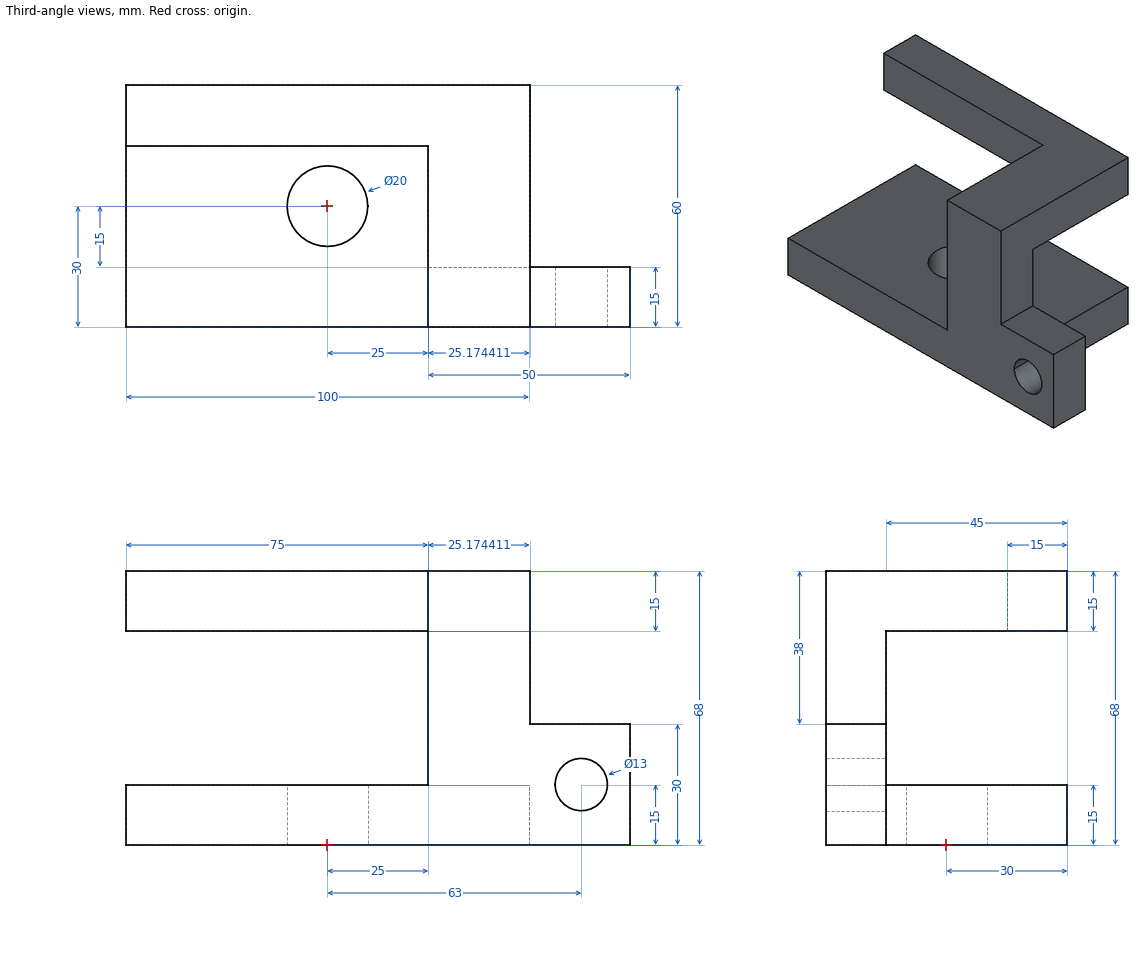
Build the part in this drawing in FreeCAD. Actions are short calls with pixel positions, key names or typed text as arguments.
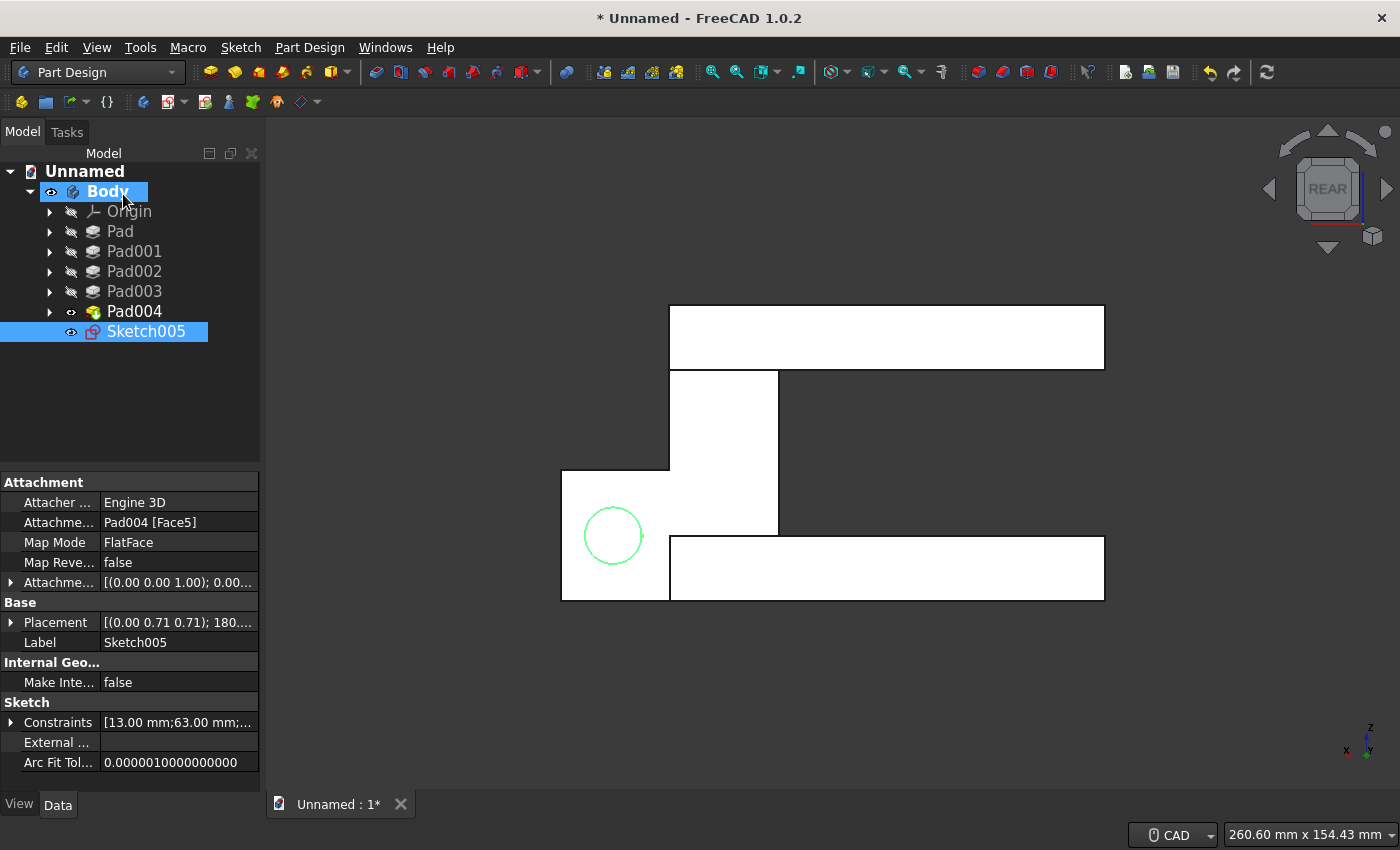
click(378, 72)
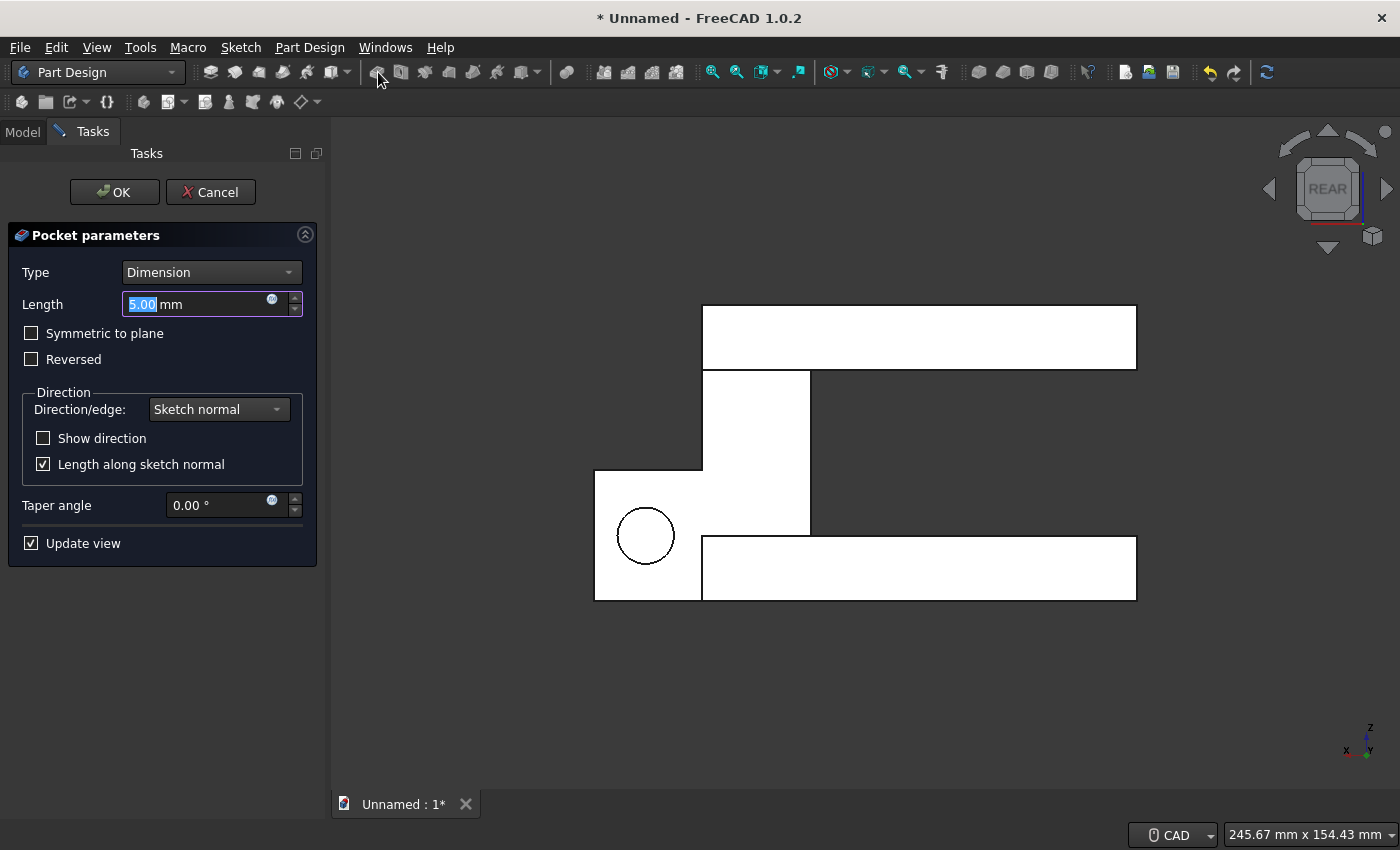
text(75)
key(Tab)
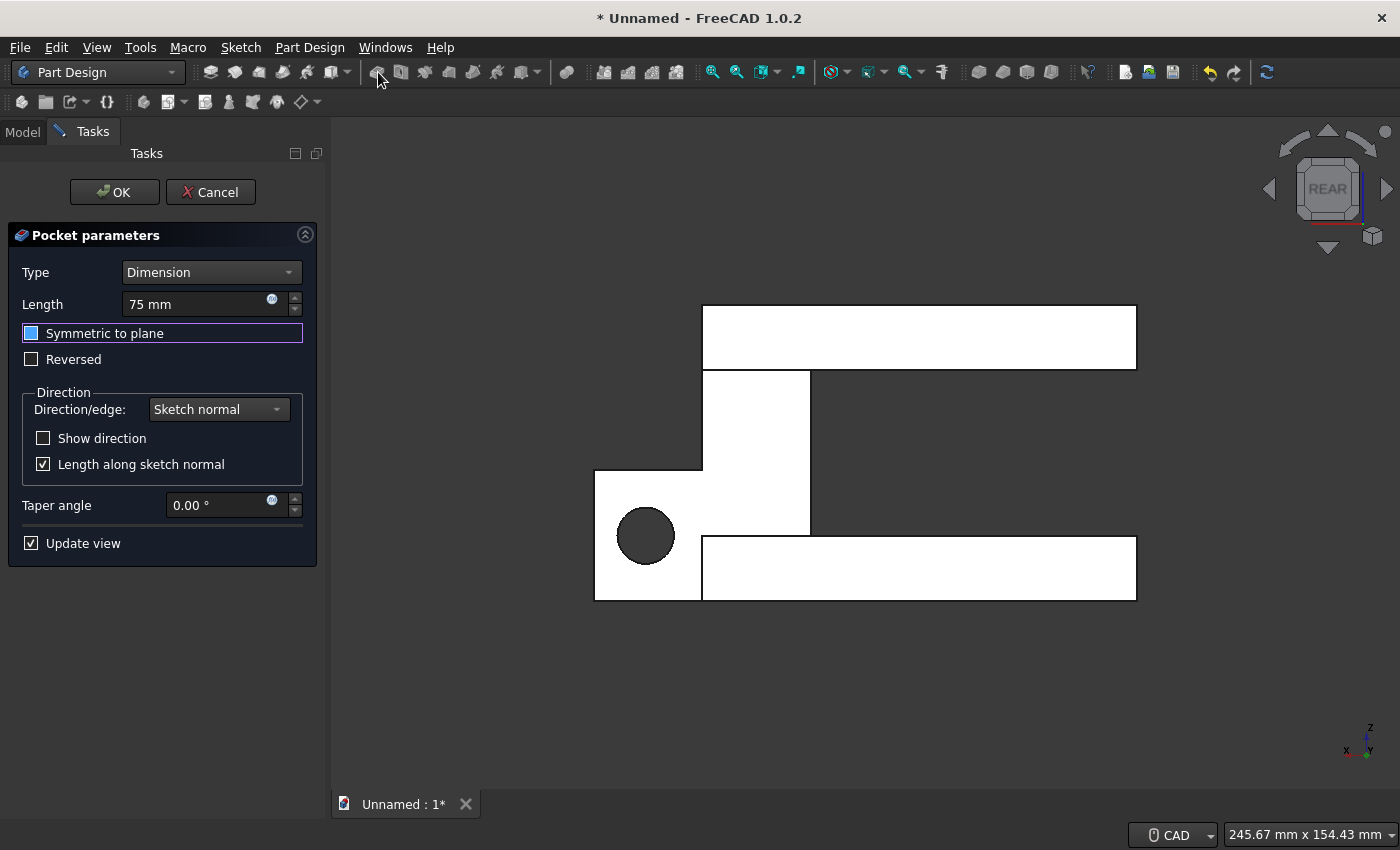
click(115, 192)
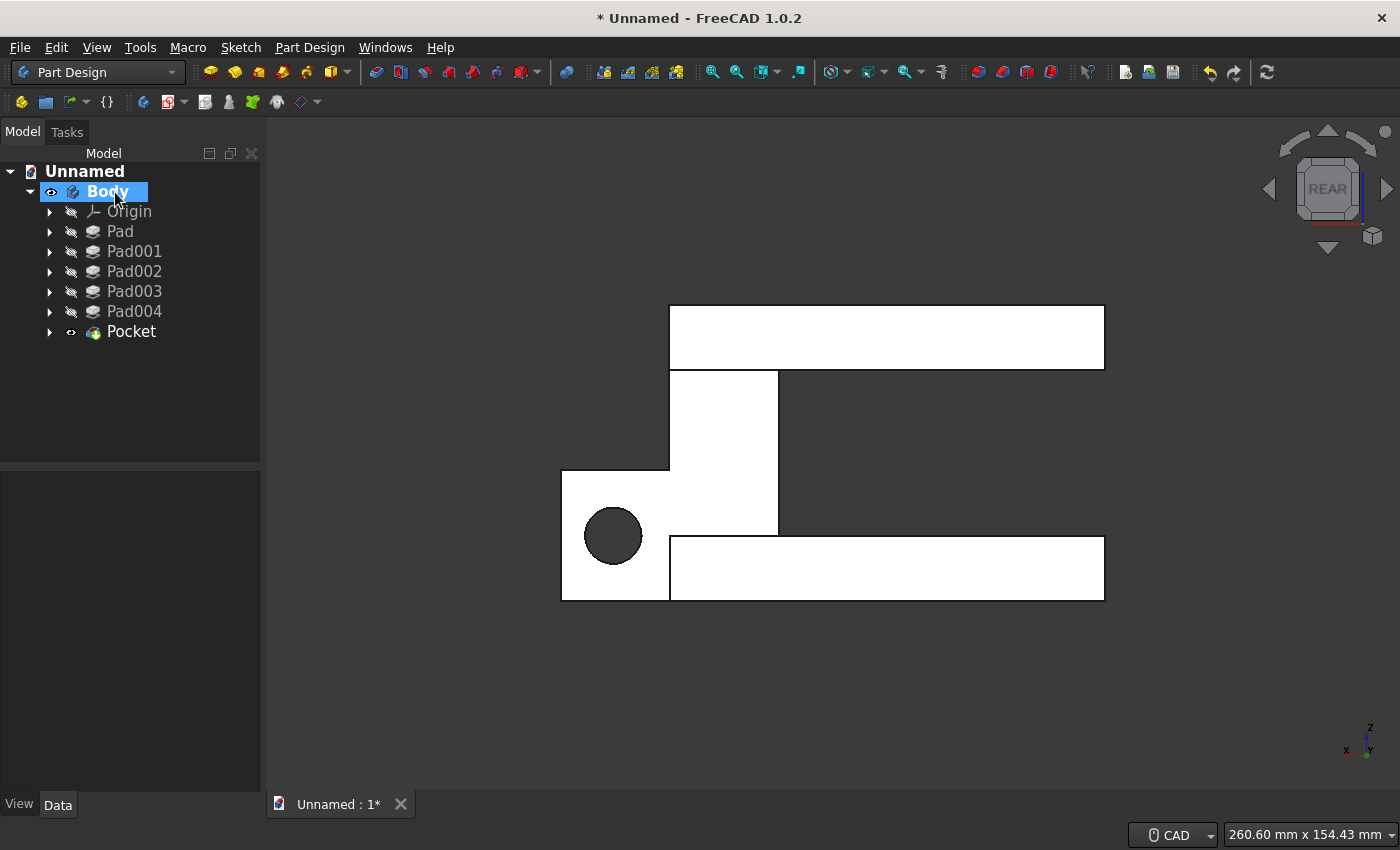
key(0)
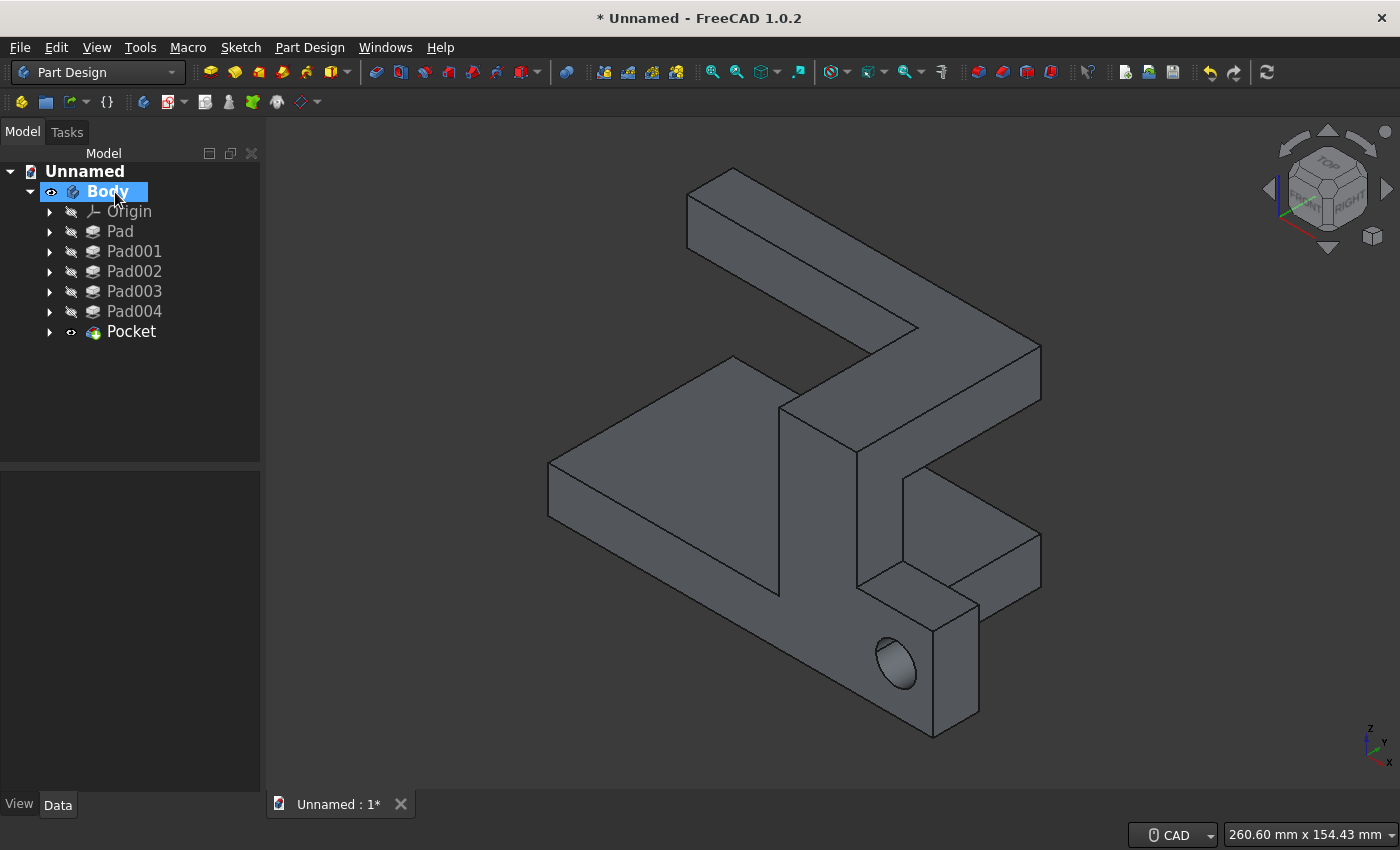
click(751, 472)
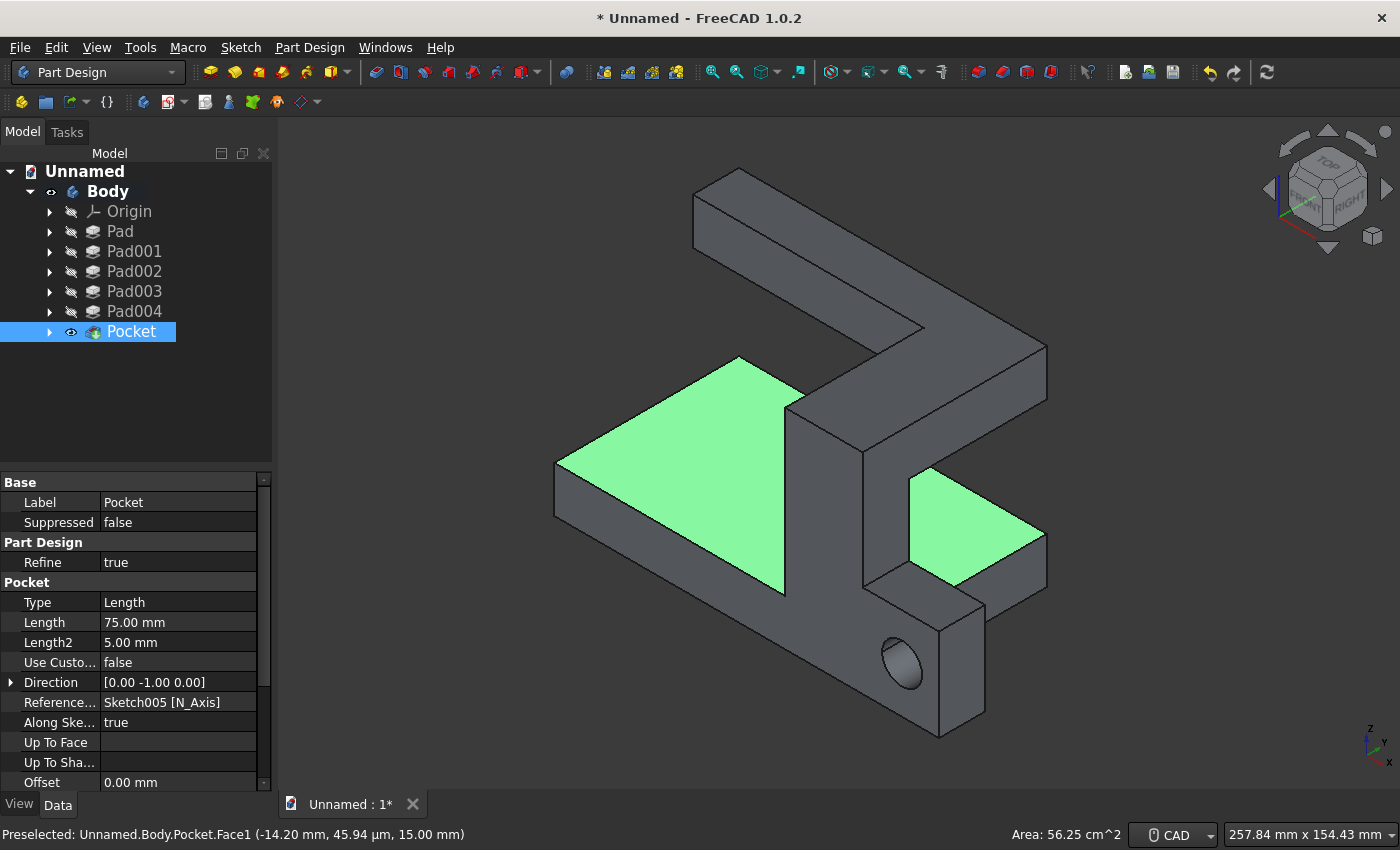
click(168, 102)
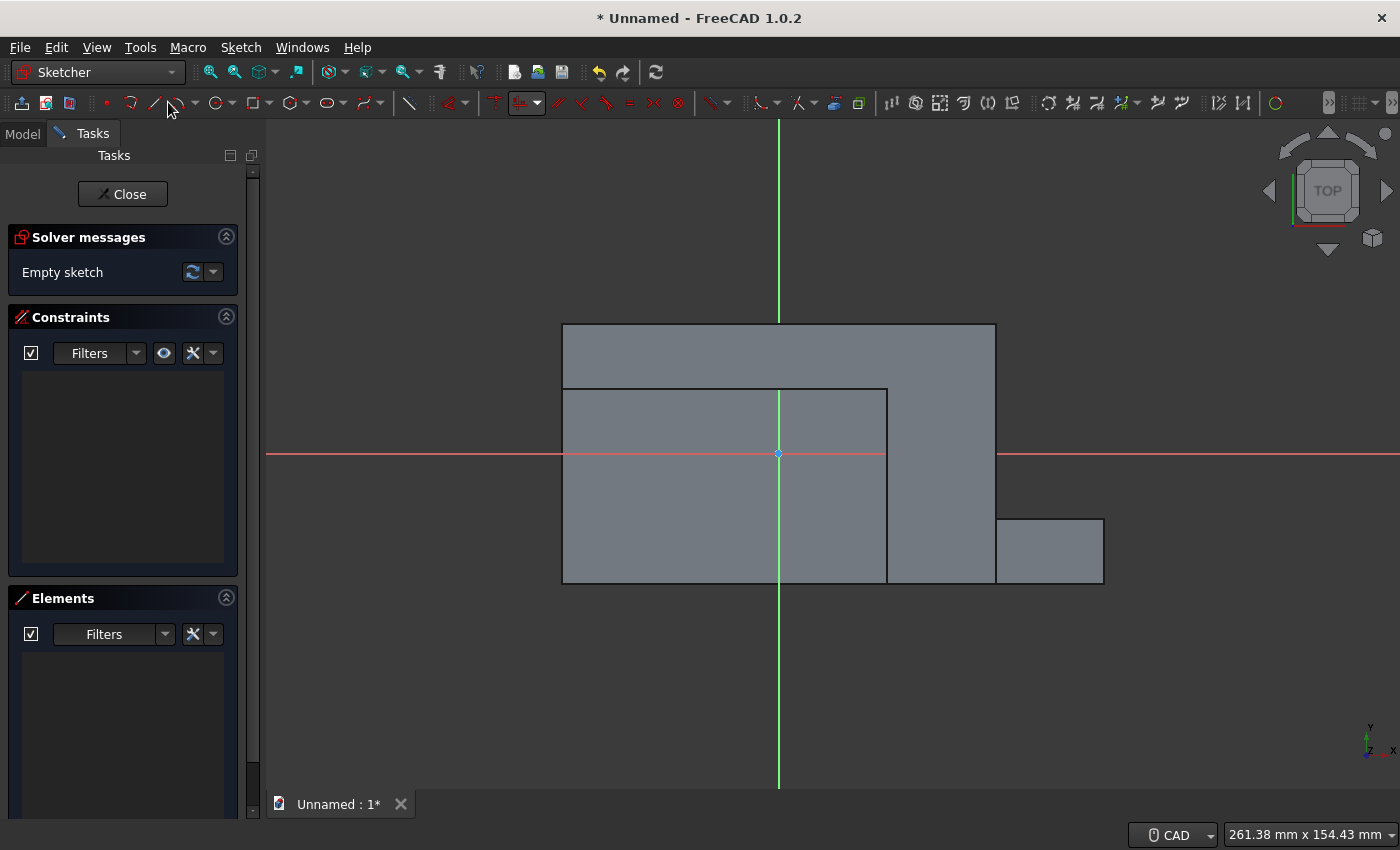
click(70, 104)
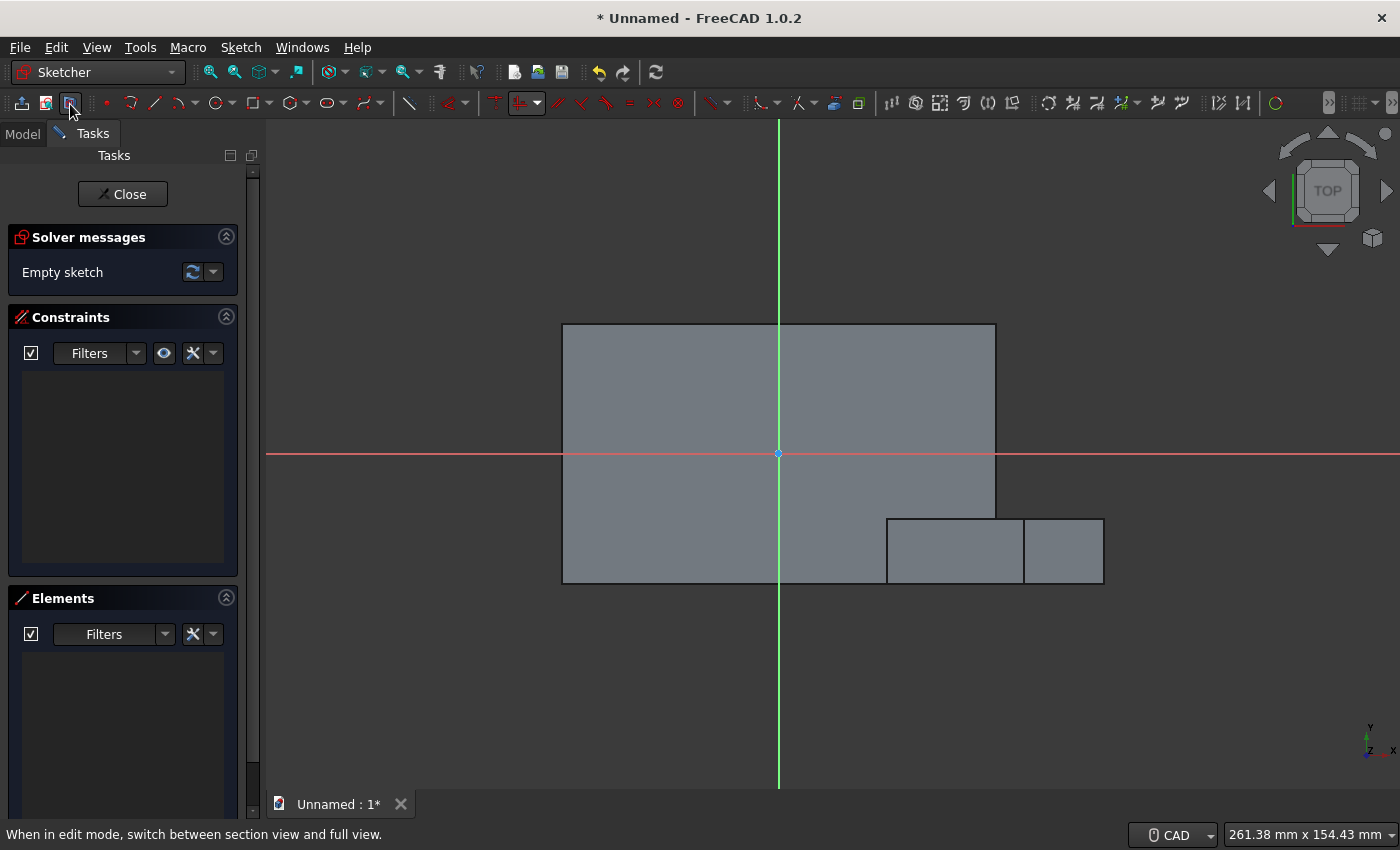
scroll(782, 454, up, 8)